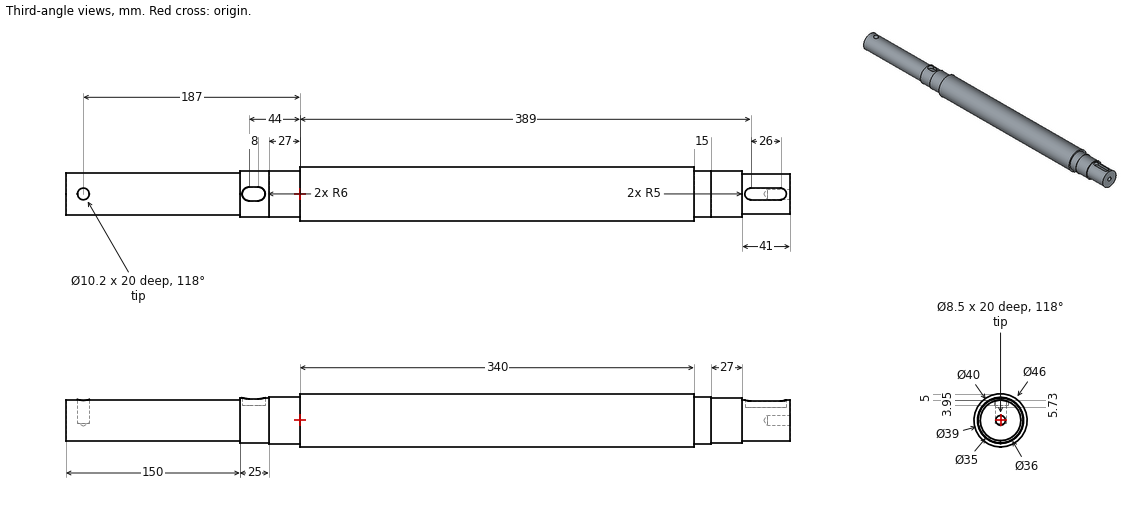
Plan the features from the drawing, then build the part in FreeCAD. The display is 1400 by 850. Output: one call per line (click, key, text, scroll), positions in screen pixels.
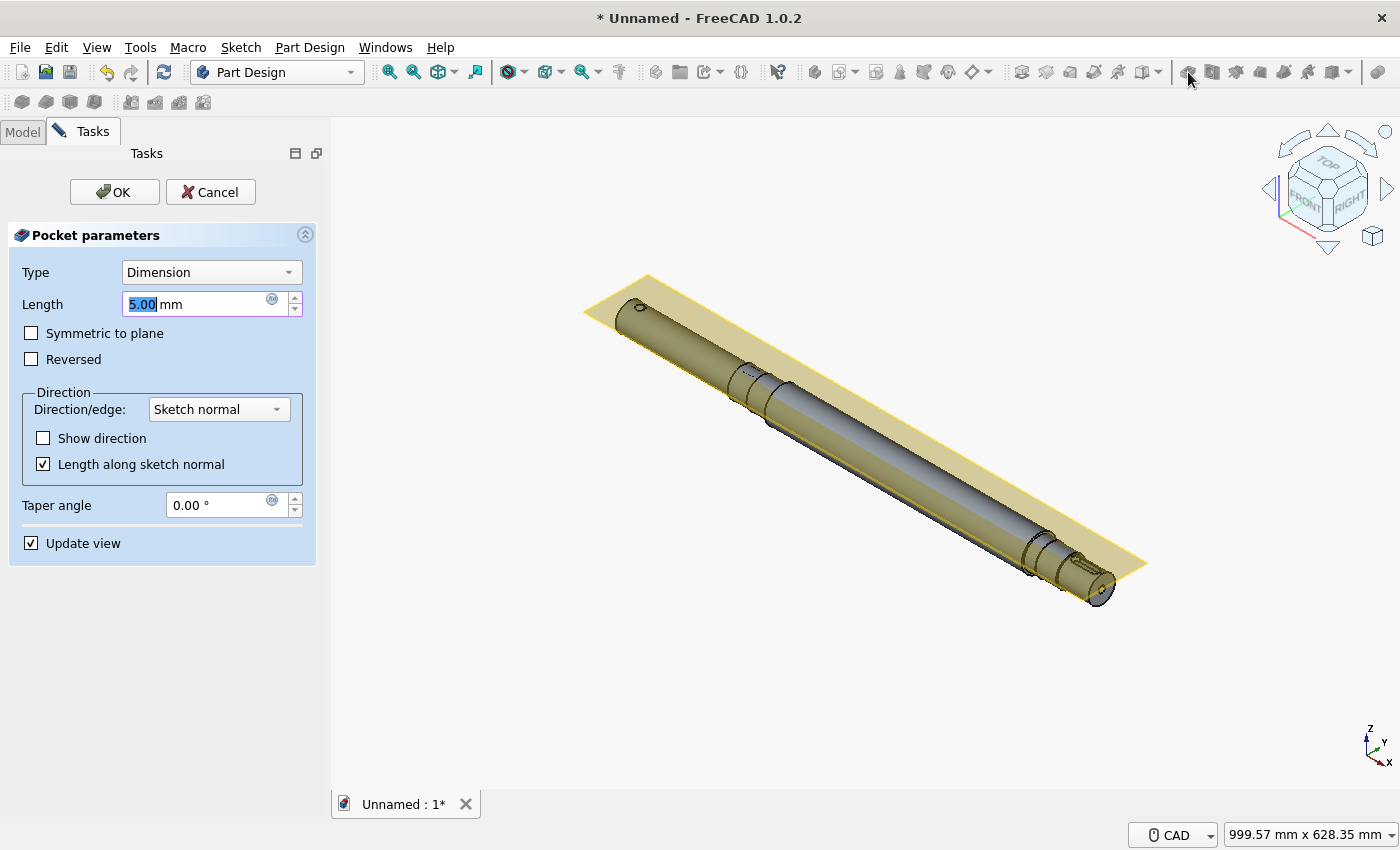
click(212, 272)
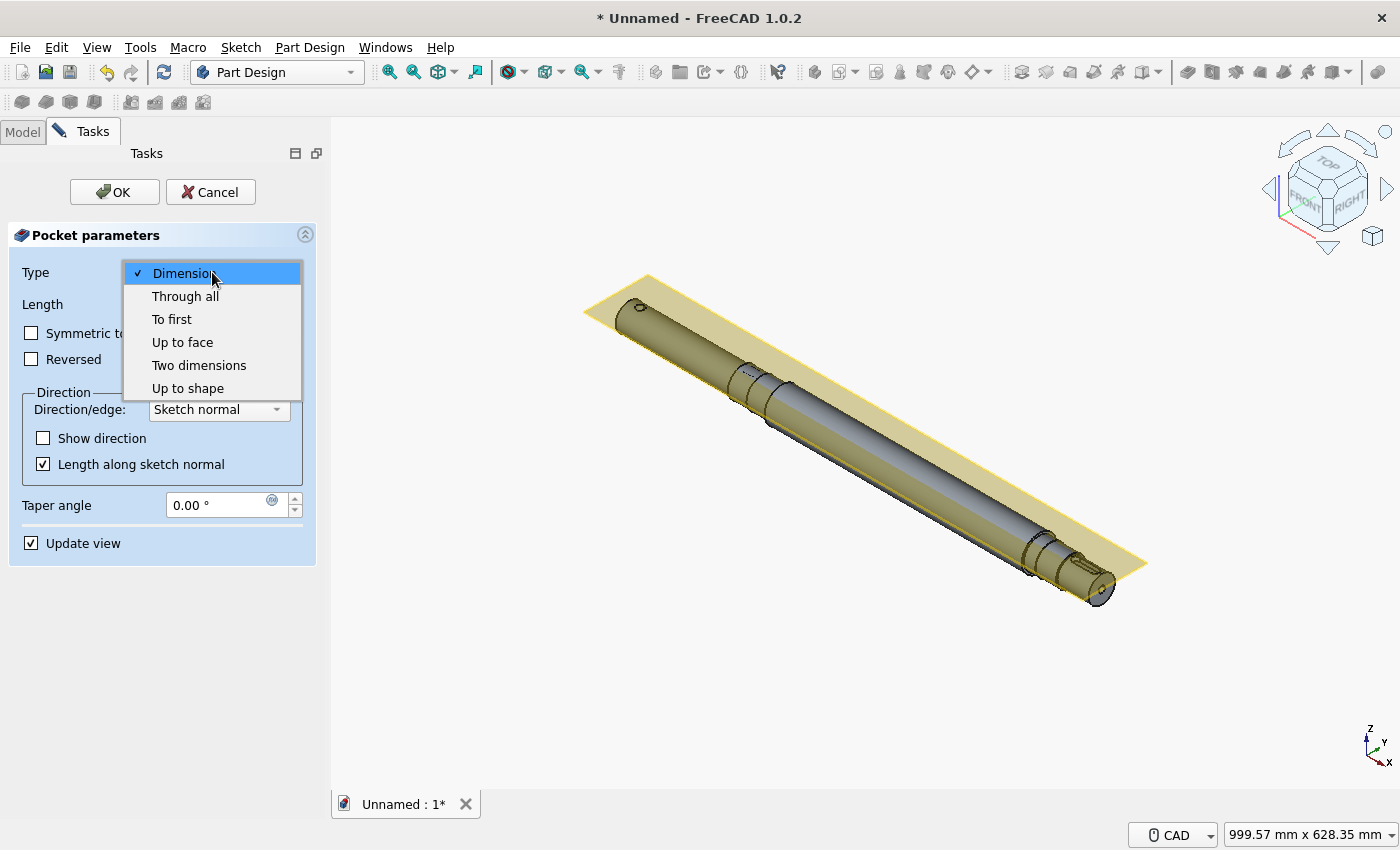
click(212, 366)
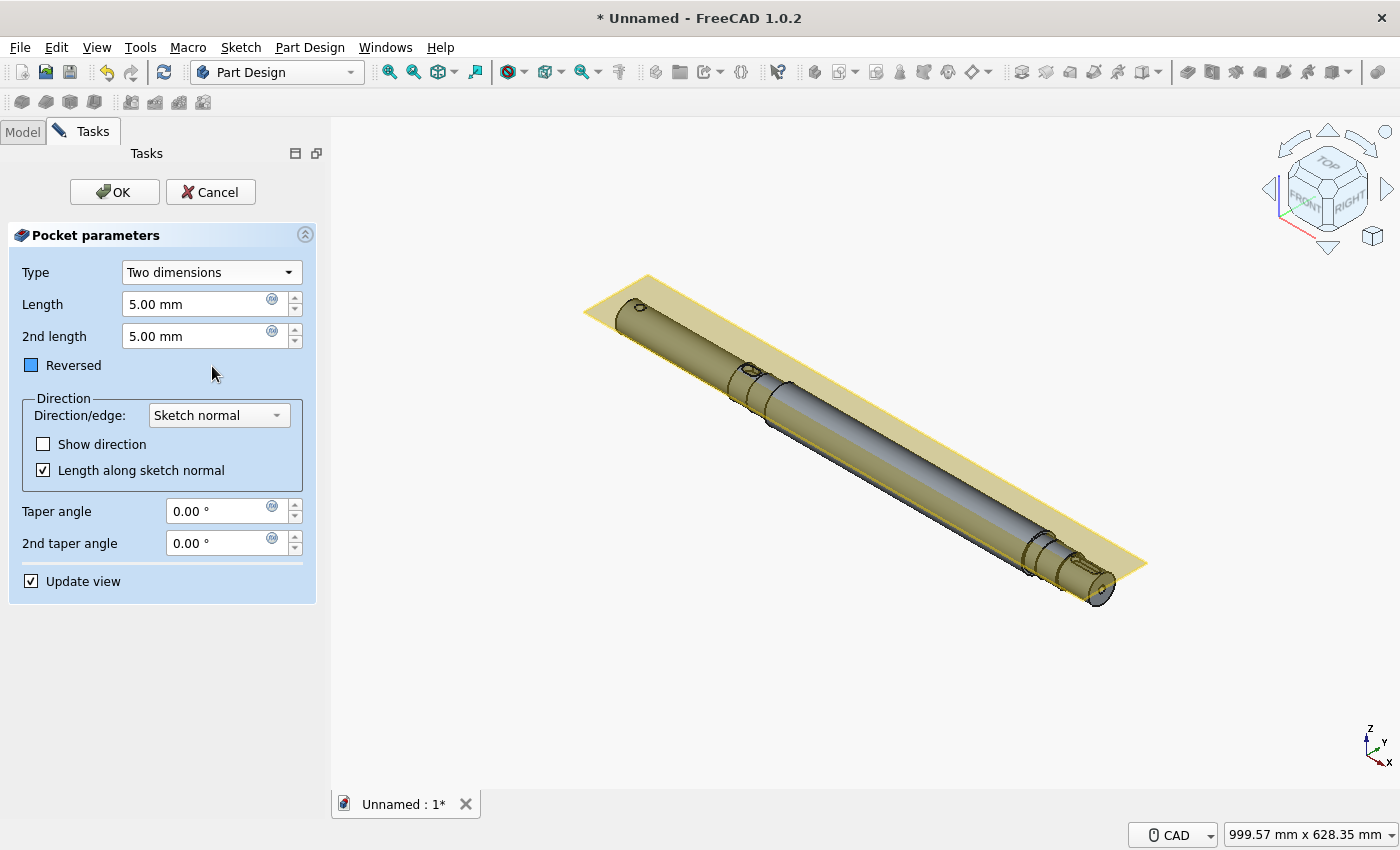
triple_click(204, 304)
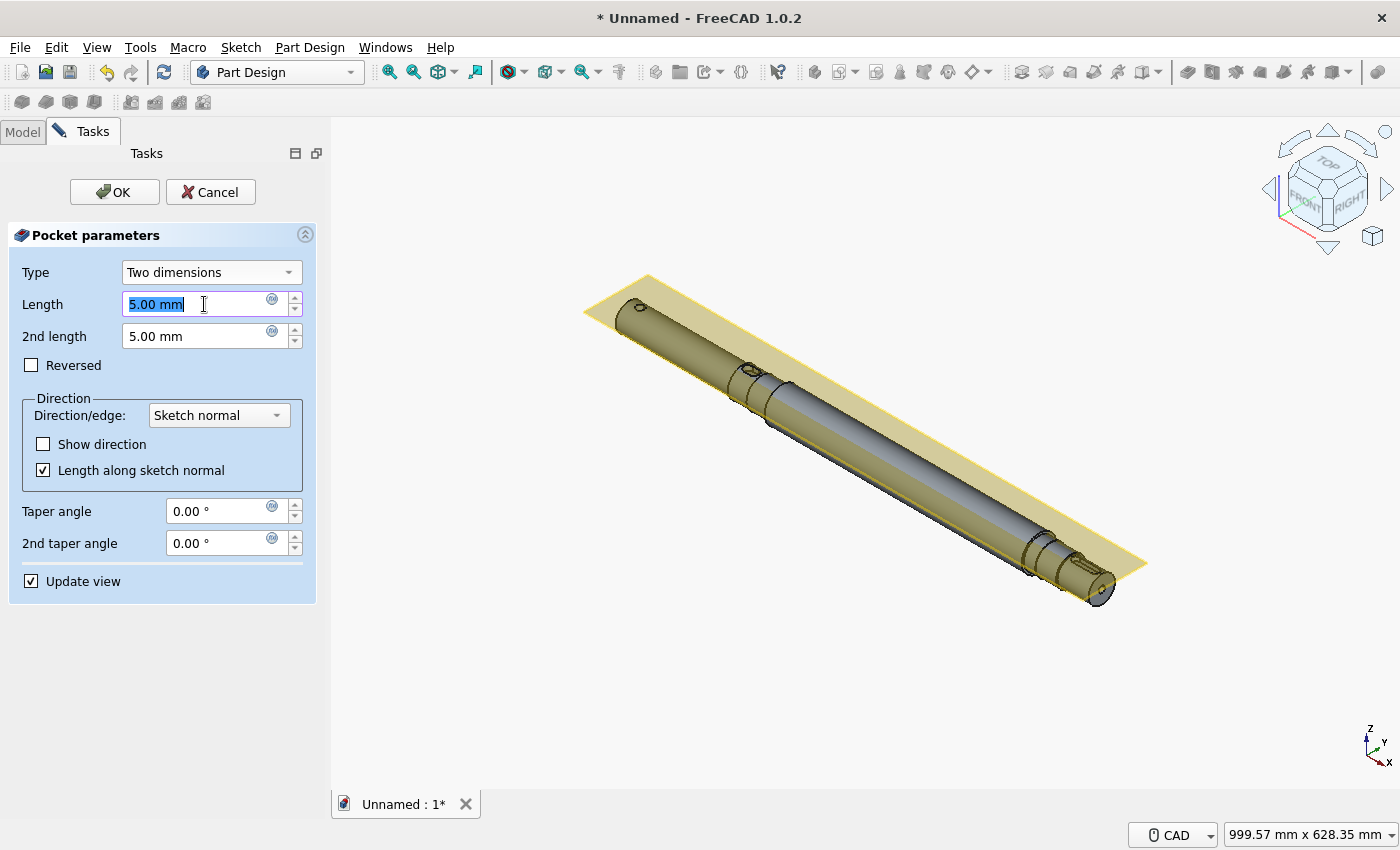
text(5)
key(Tab)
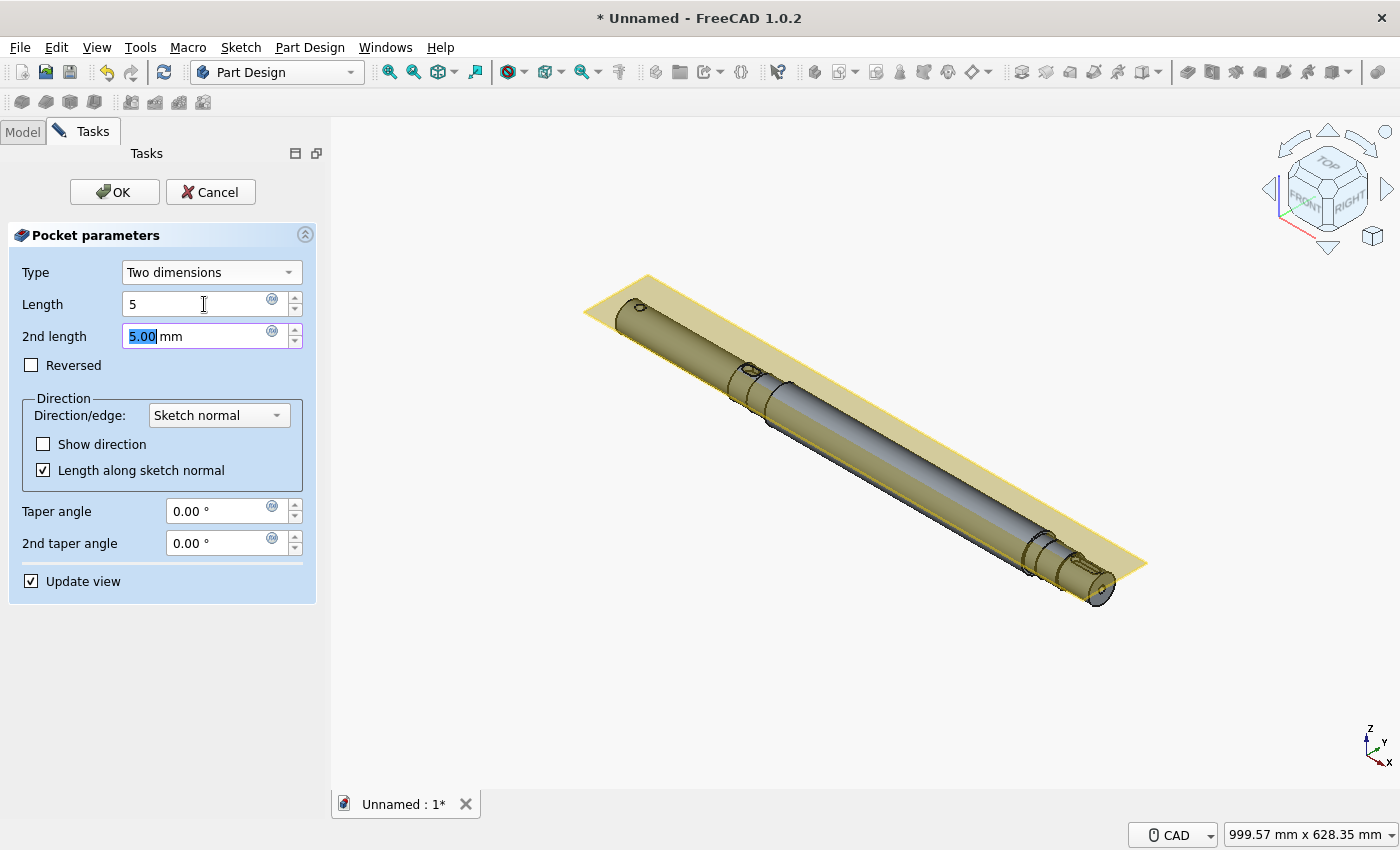
text(3.95)
key(Tab)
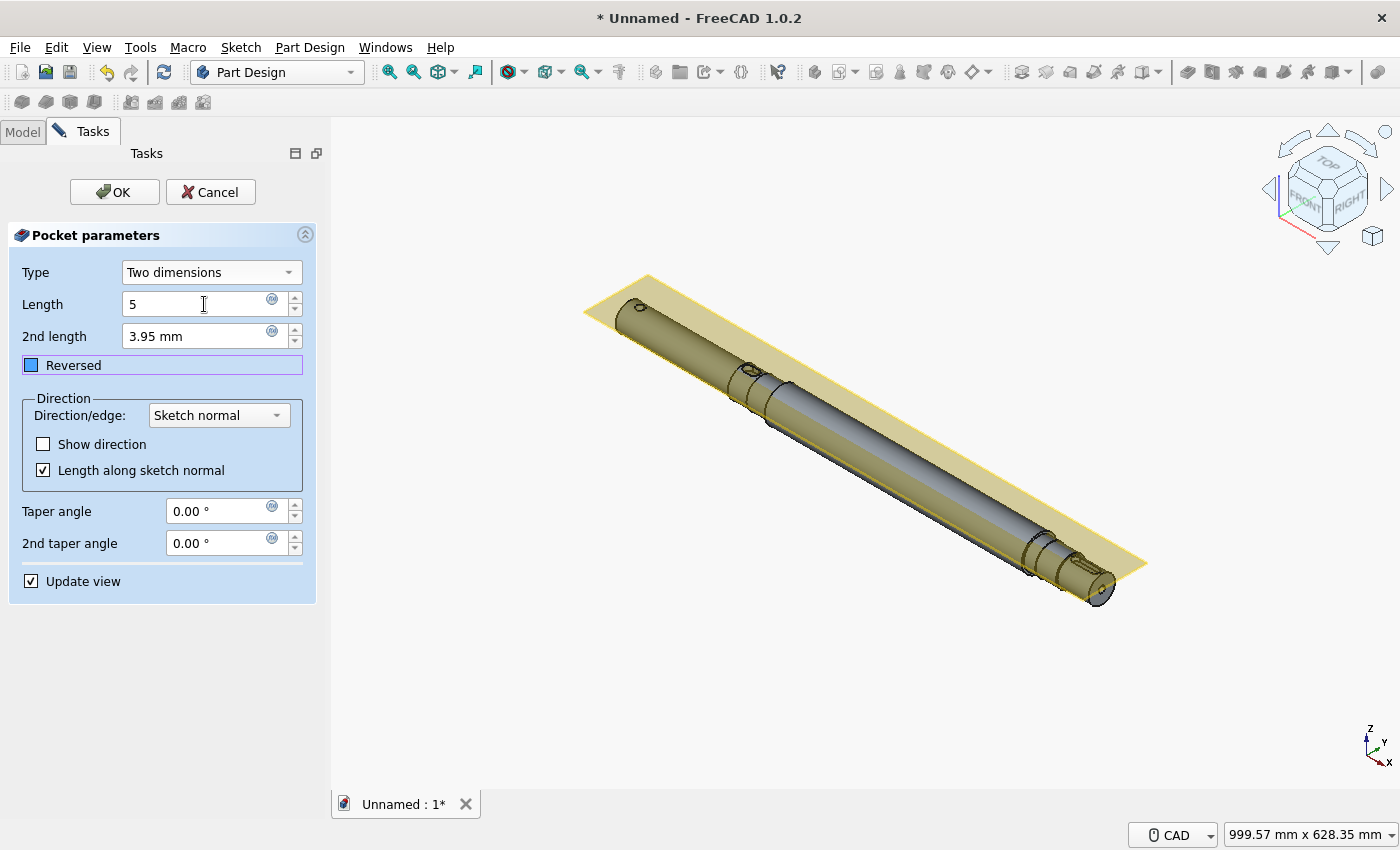
click(30, 365)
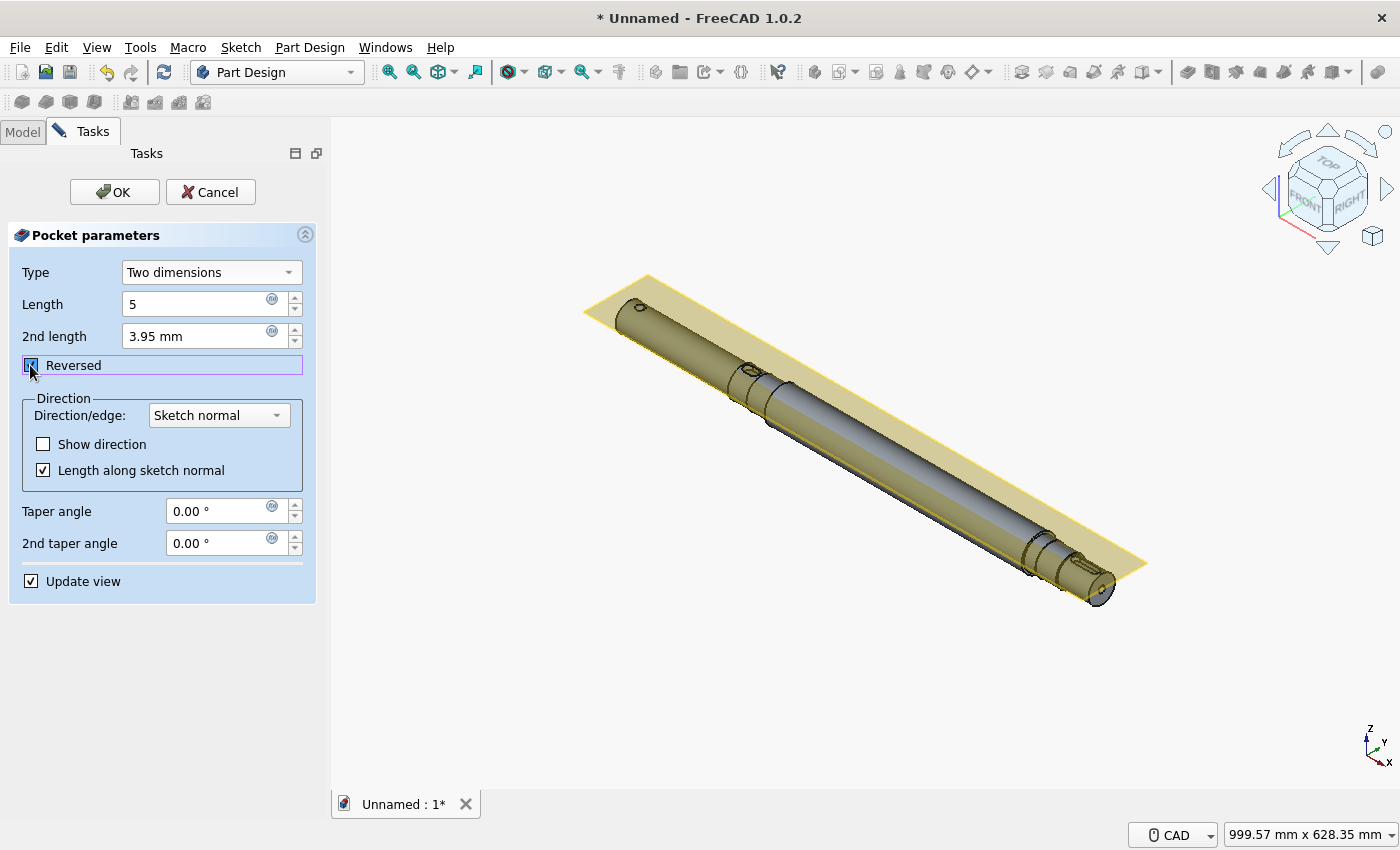
click(115, 192)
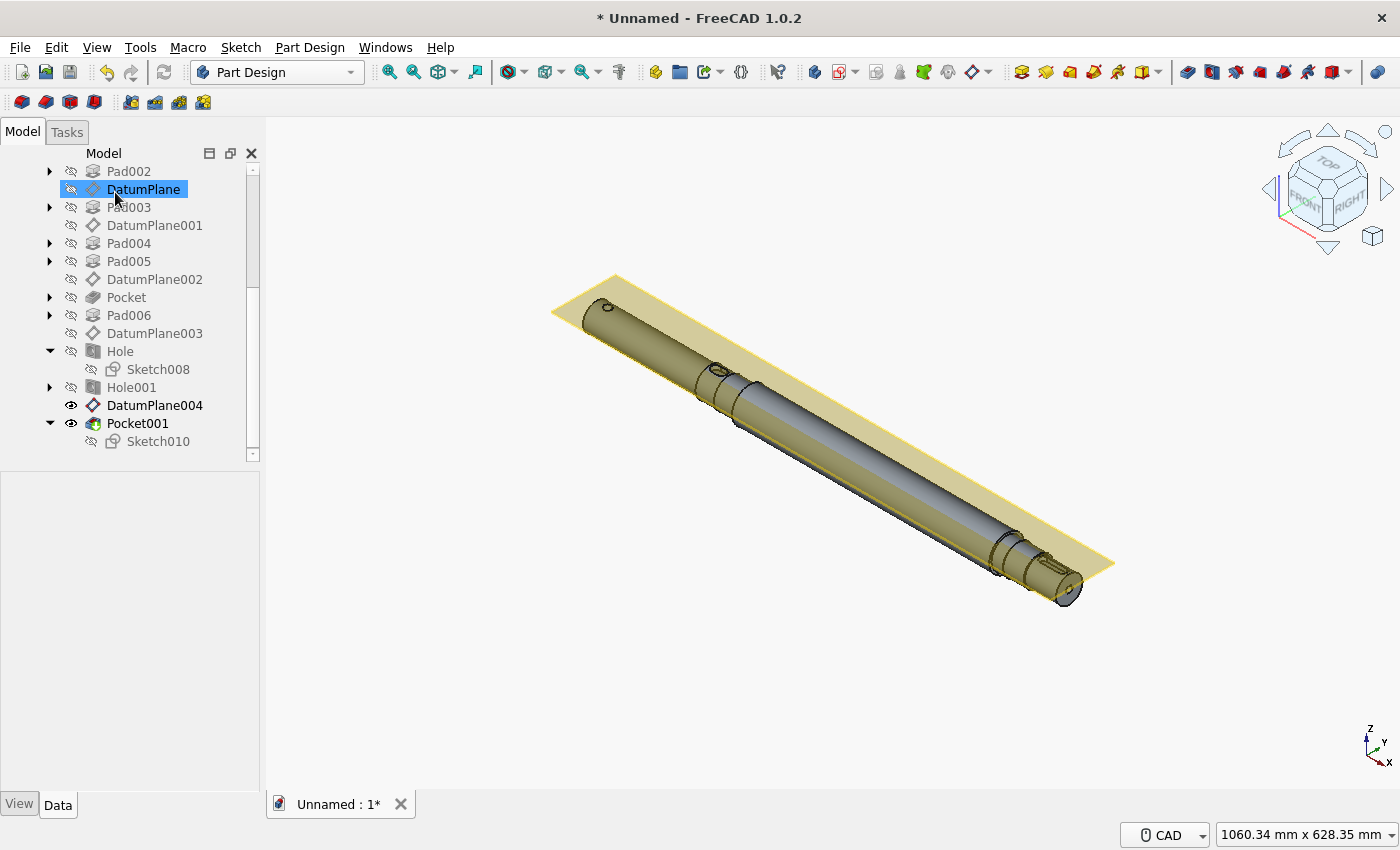
click(116, 405)
key(space)